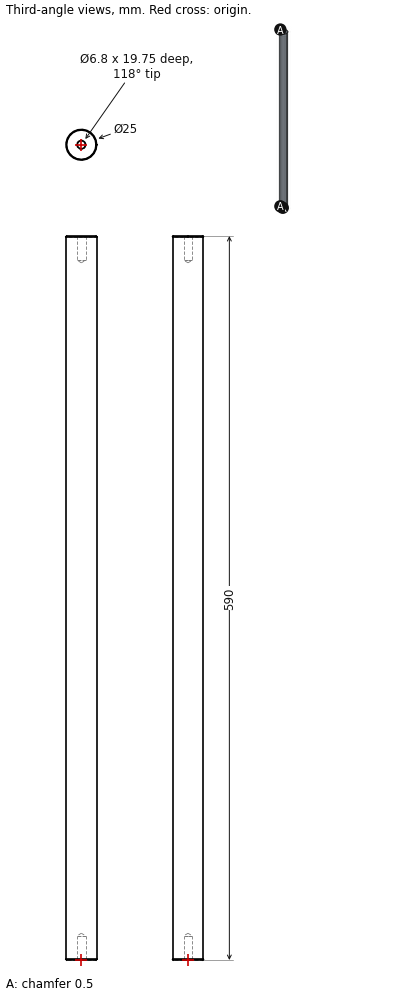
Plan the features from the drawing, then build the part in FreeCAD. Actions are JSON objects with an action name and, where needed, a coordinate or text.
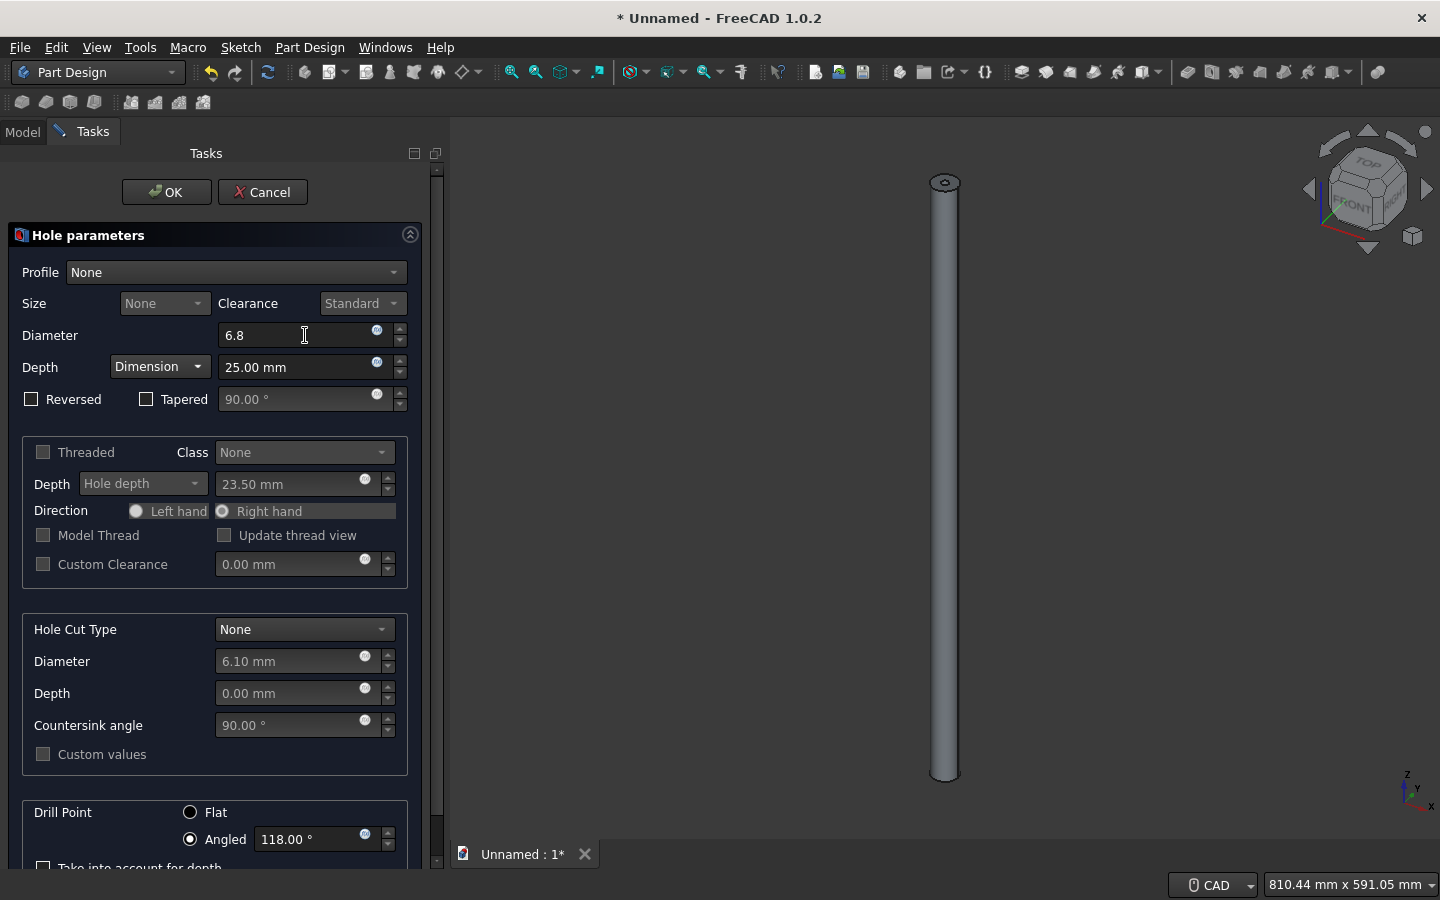
{"action": "triple_click", "coordinate": [305, 367]}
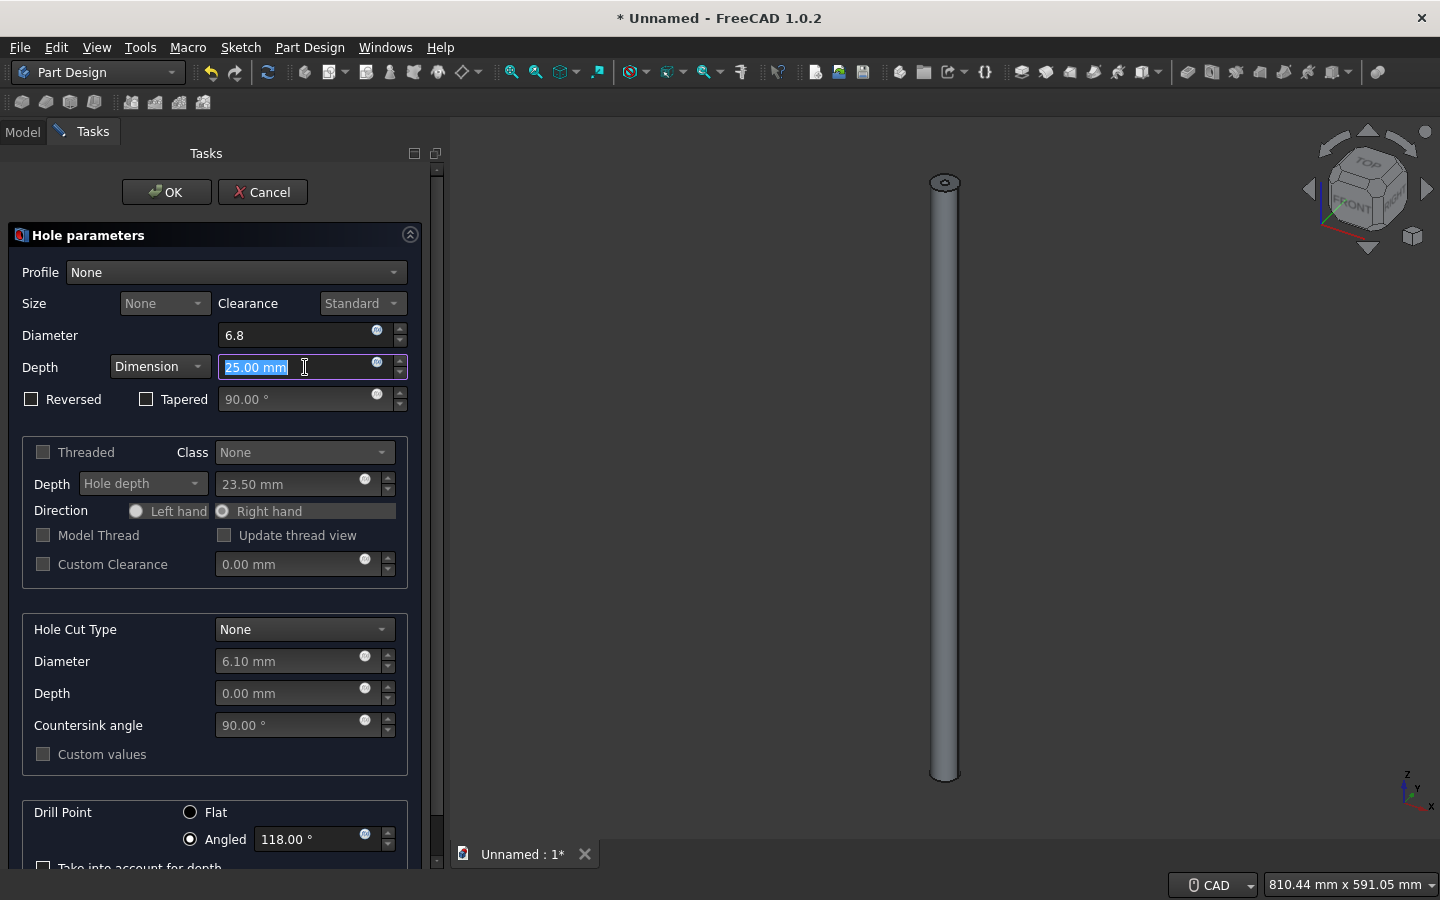
{"action": "type", "text": "19.75"}
{"action": "key", "text": "Tab"}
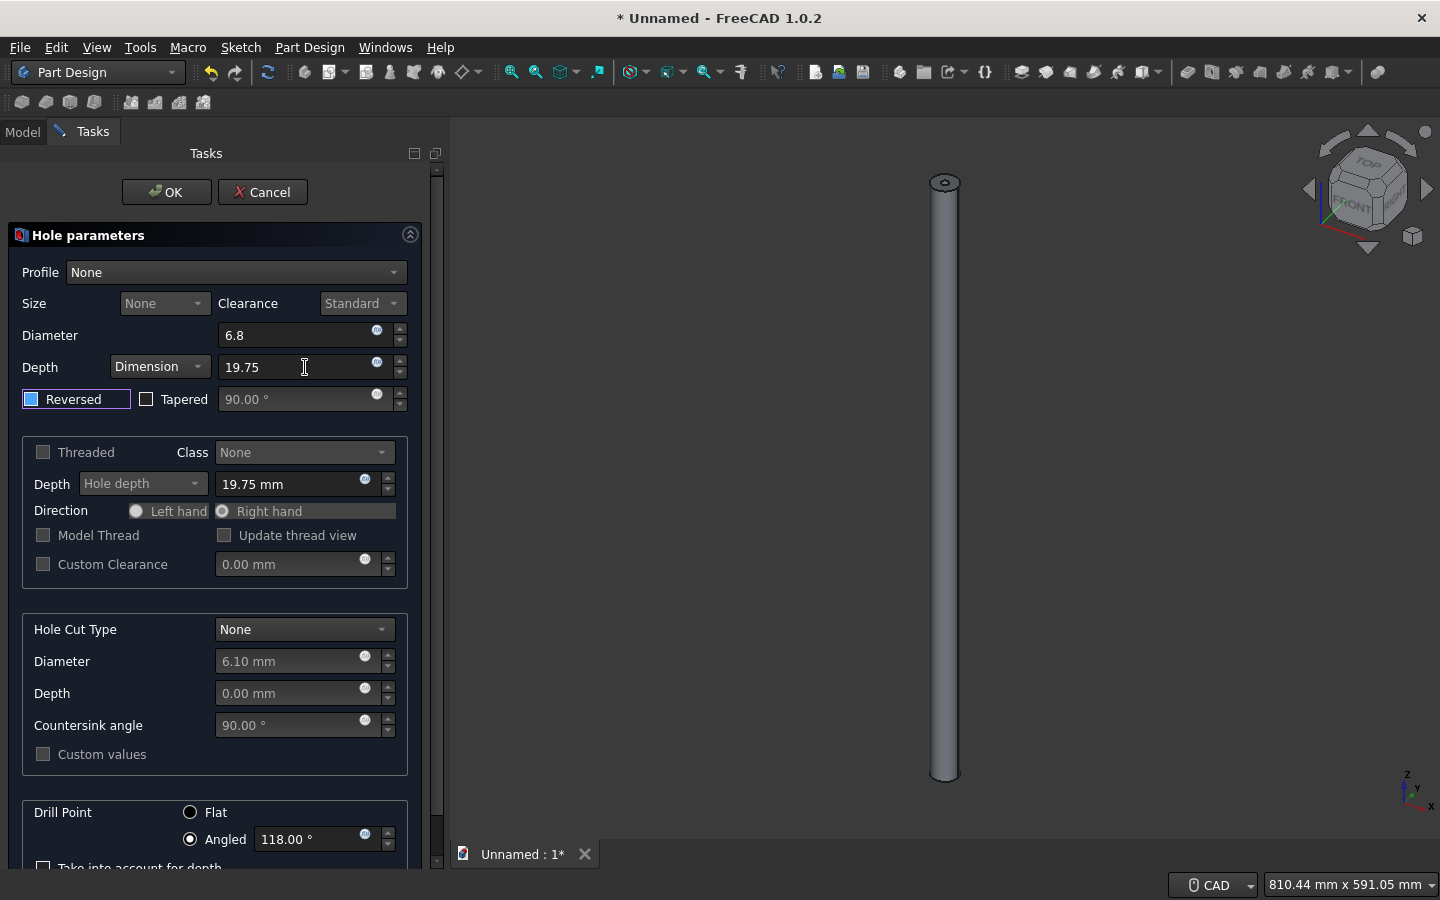
{"action": "left_click", "coordinate": [167, 192]}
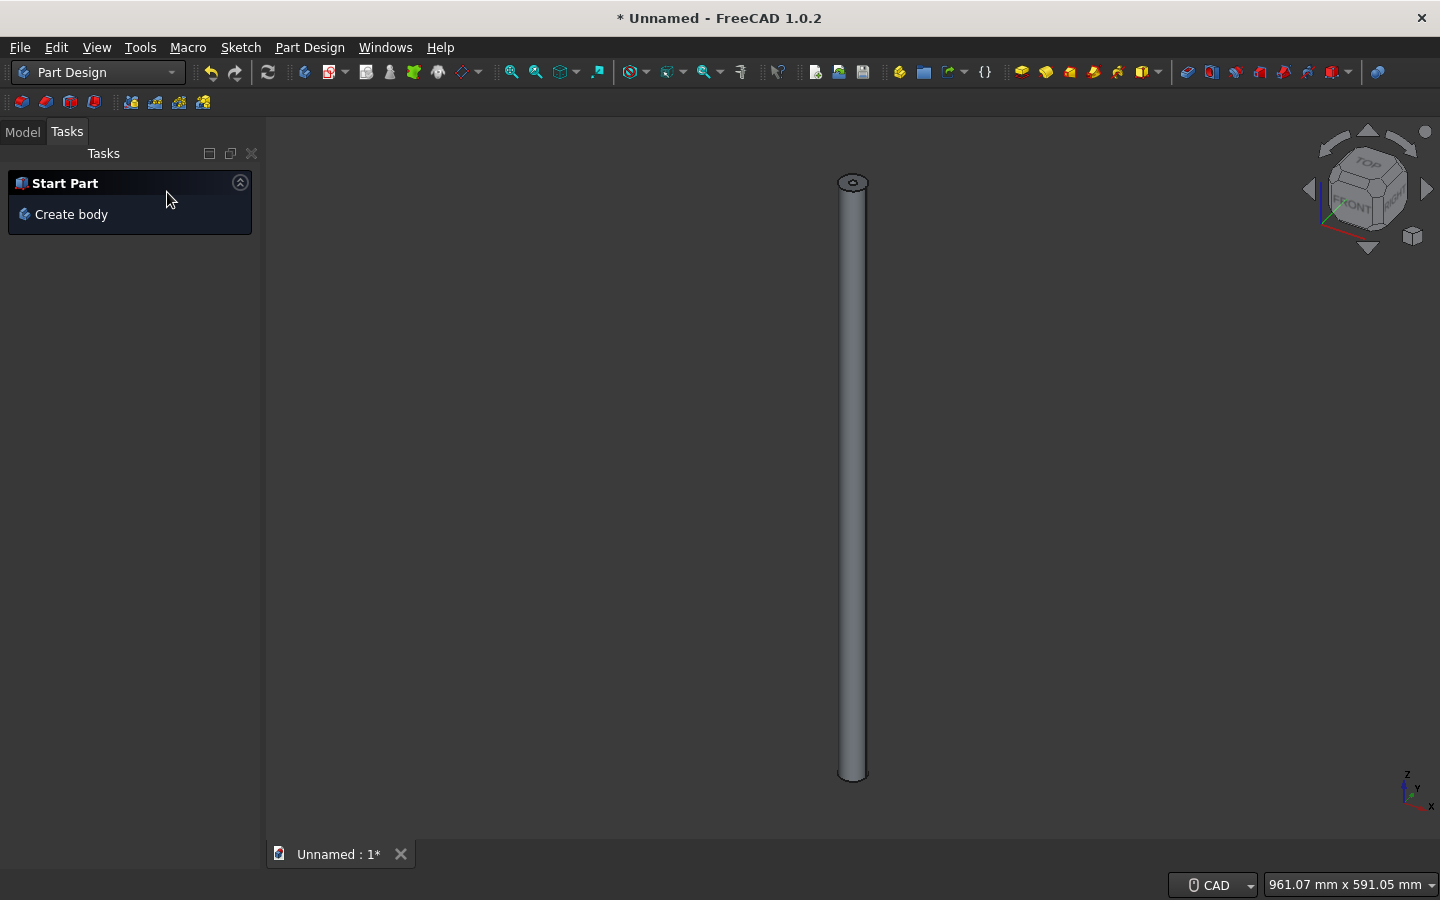
{"action": "key", "text": "5"}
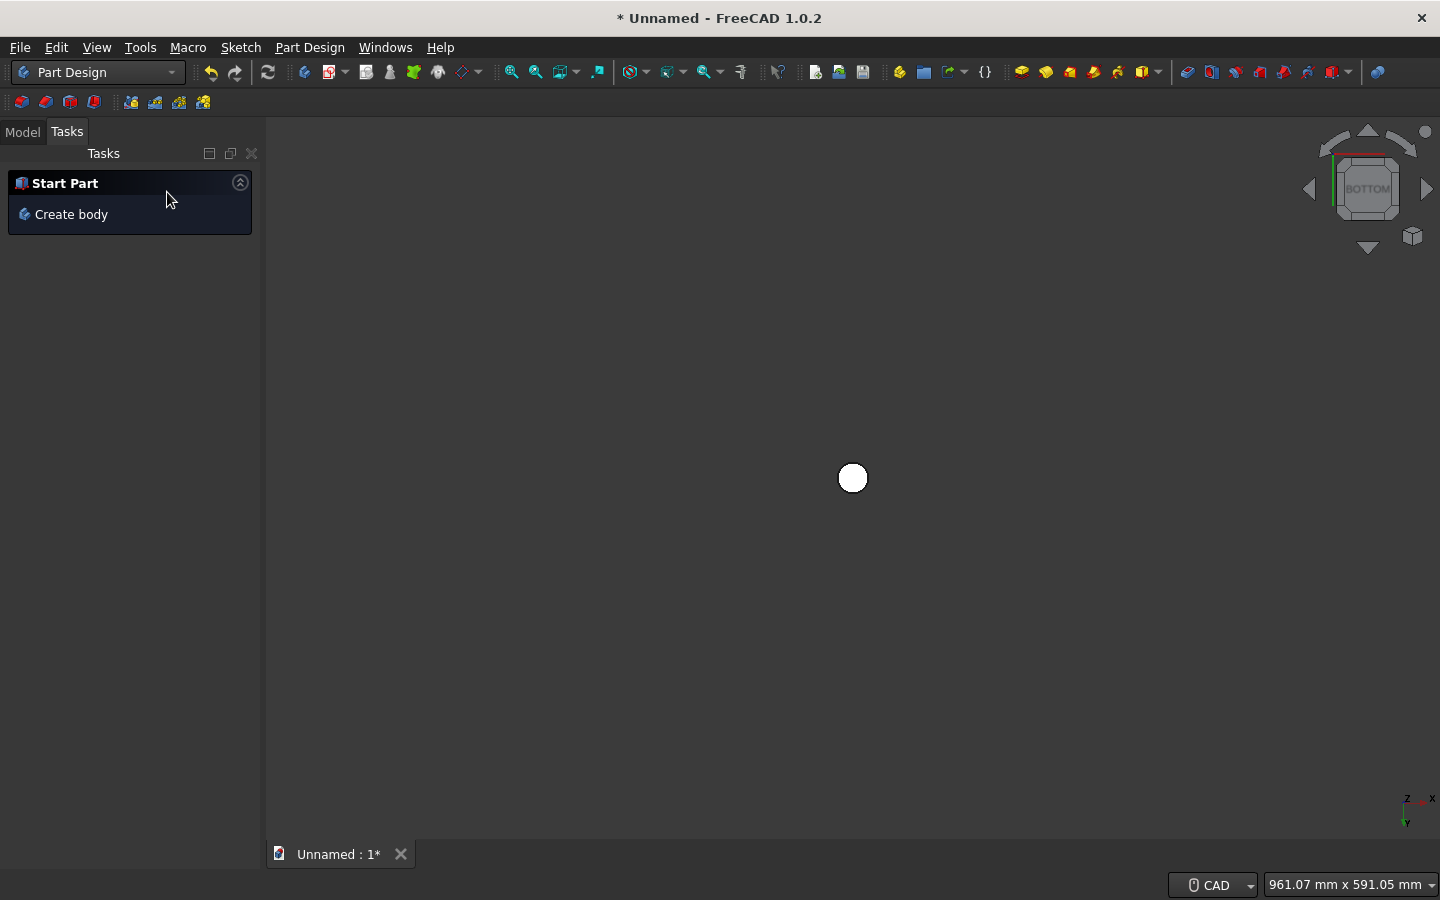
{"action": "key", "text": "v f"}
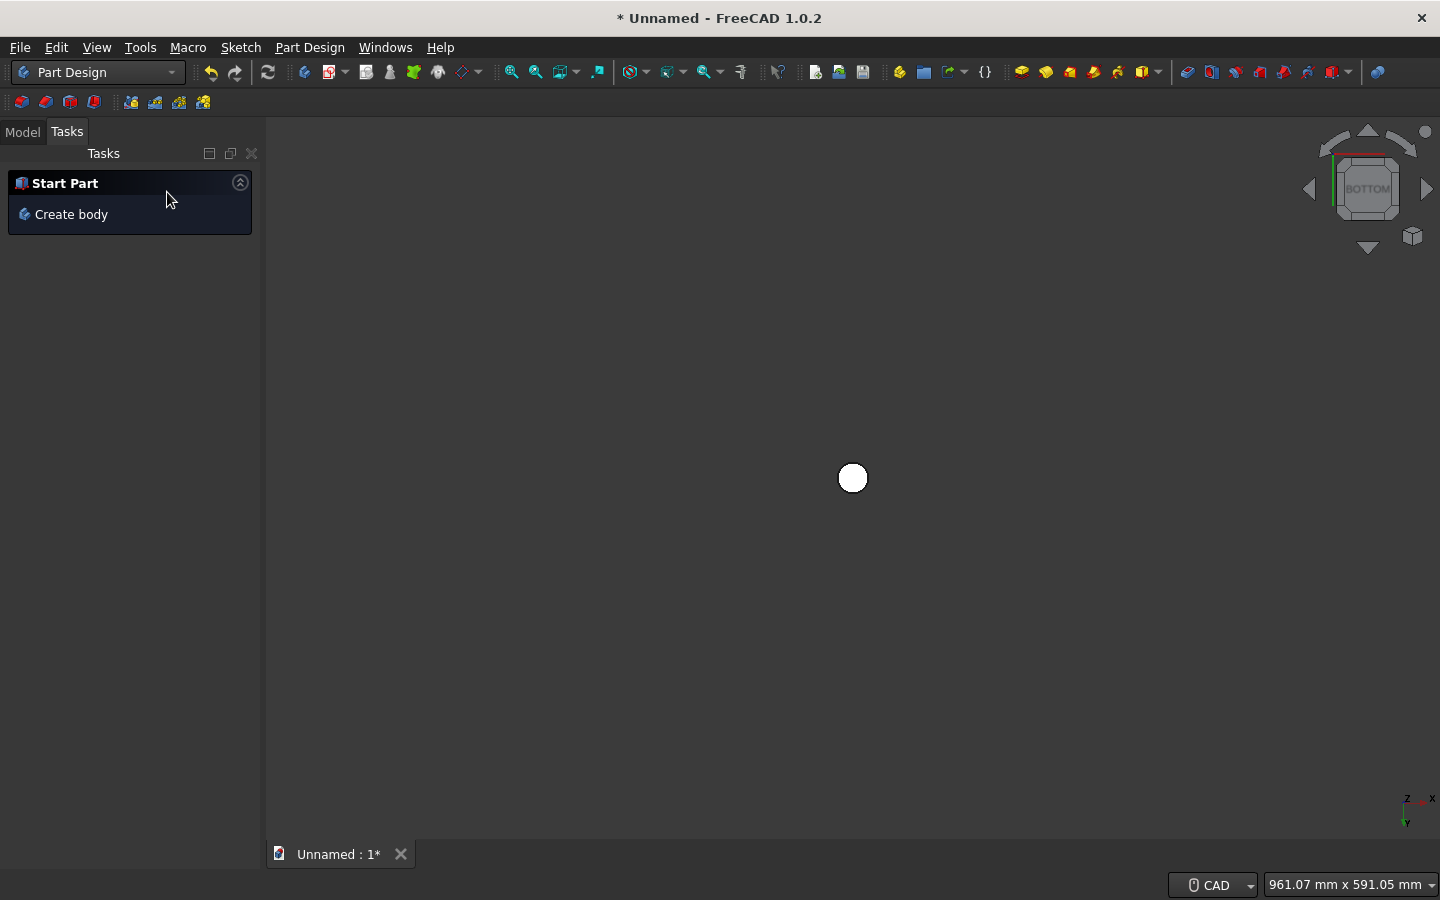
{"action": "left_click", "coordinate": [853, 477]}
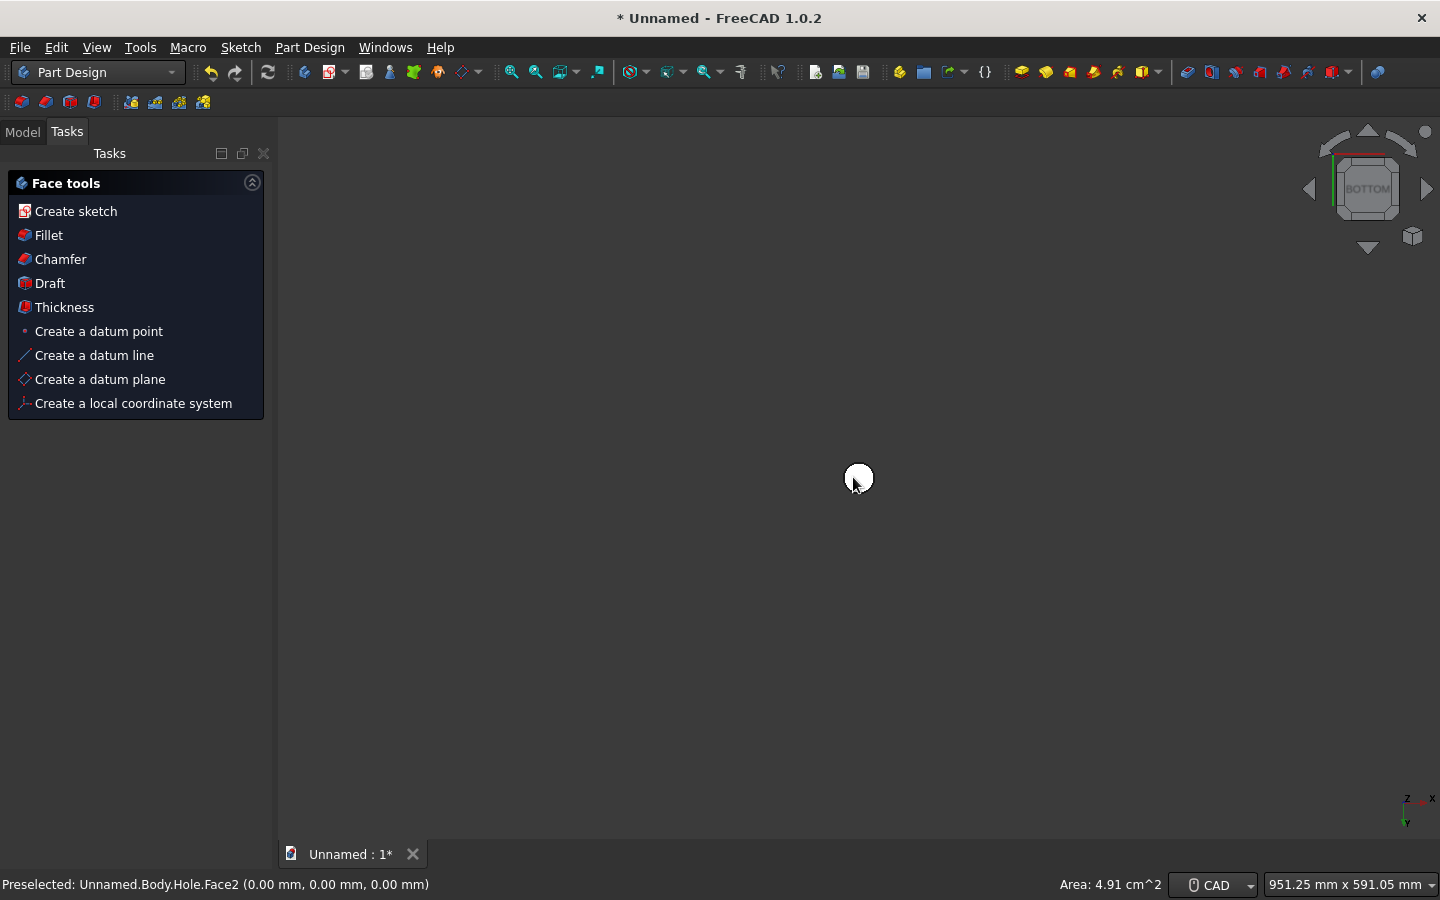
{"action": "left_click", "coordinate": [330, 72]}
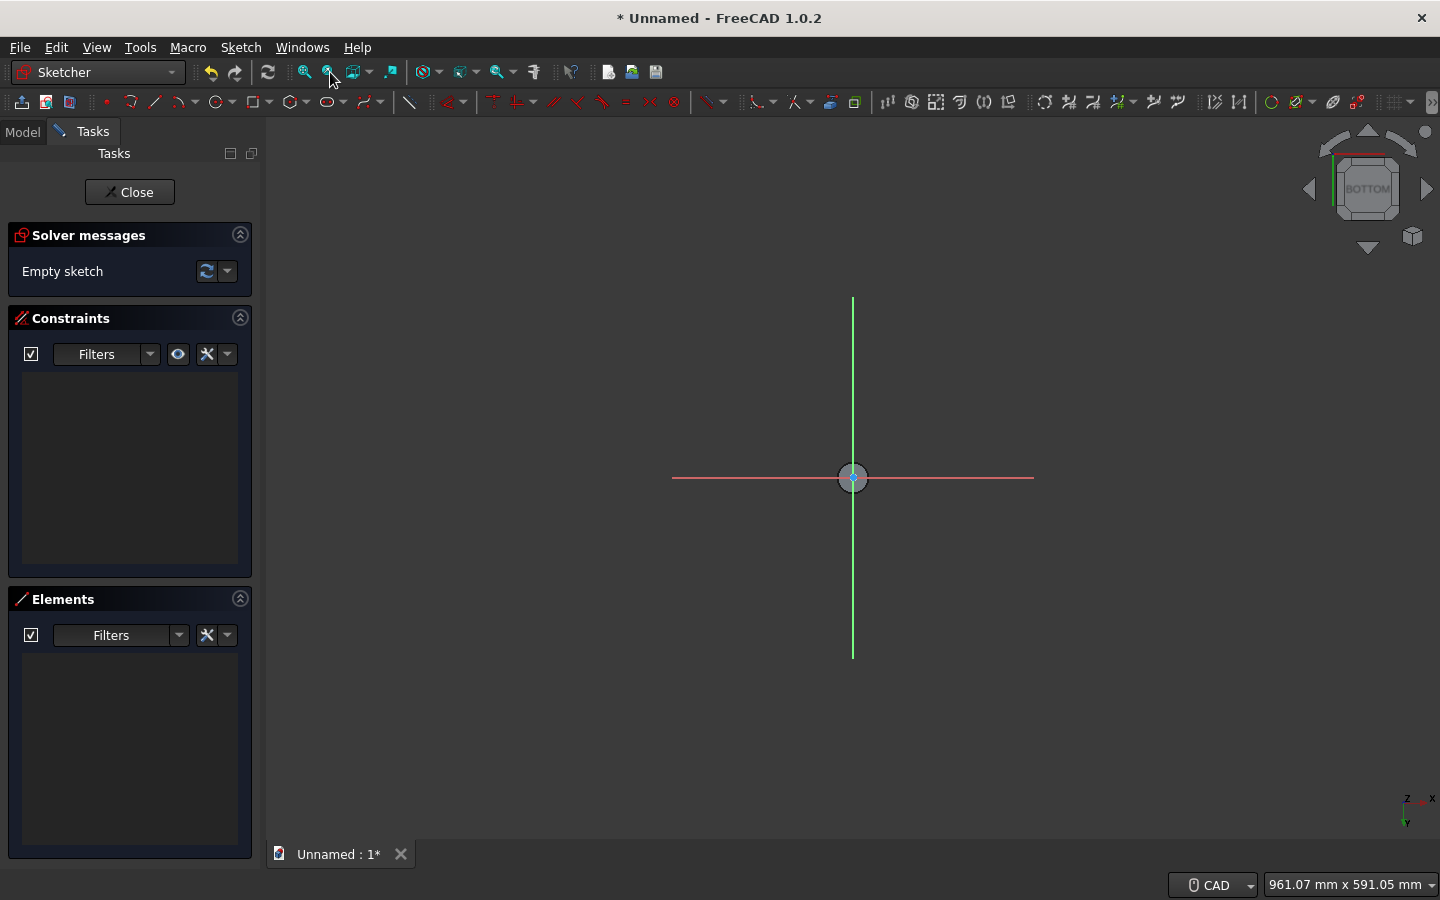
{"action": "scroll", "coordinate": [857, 478], "scroll_direction": "up", "scroll_amount": 15}